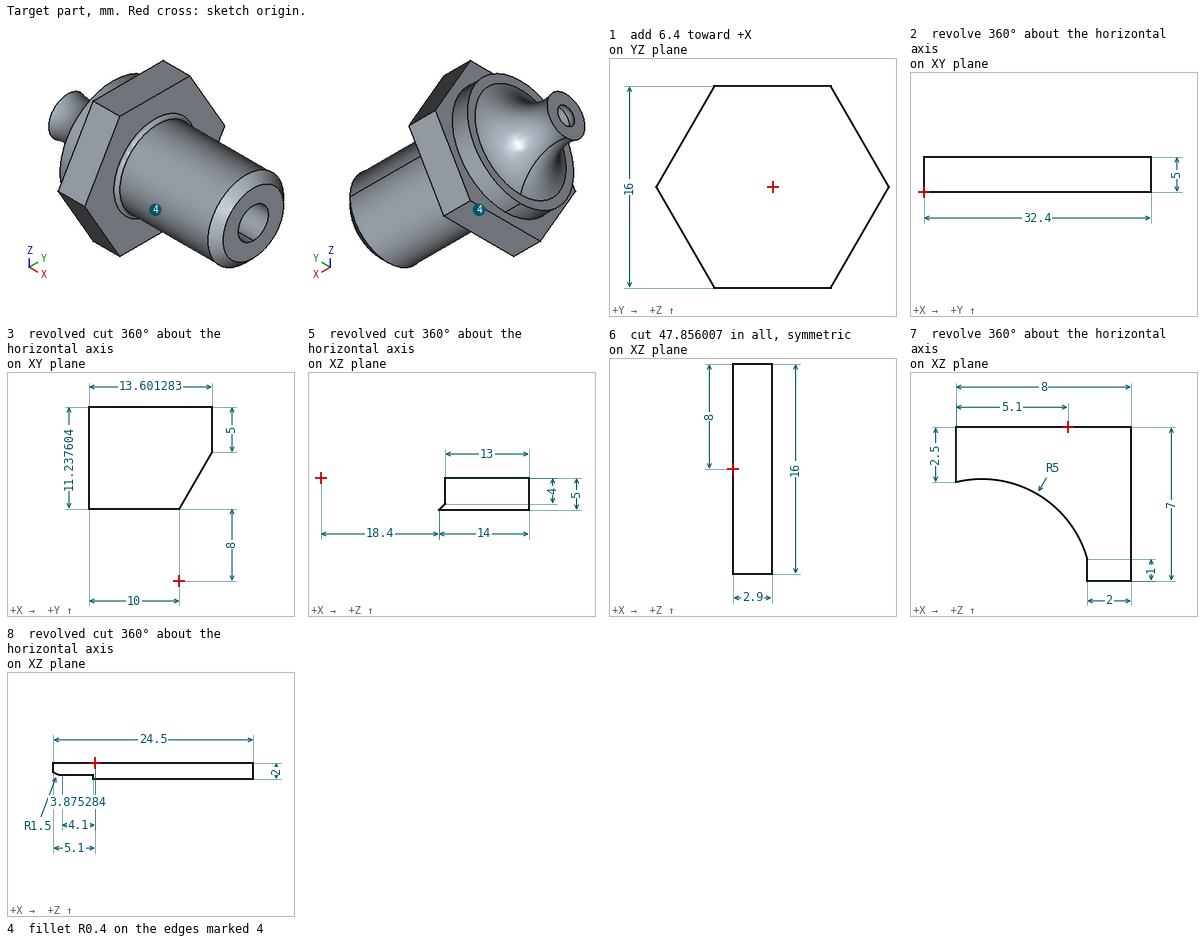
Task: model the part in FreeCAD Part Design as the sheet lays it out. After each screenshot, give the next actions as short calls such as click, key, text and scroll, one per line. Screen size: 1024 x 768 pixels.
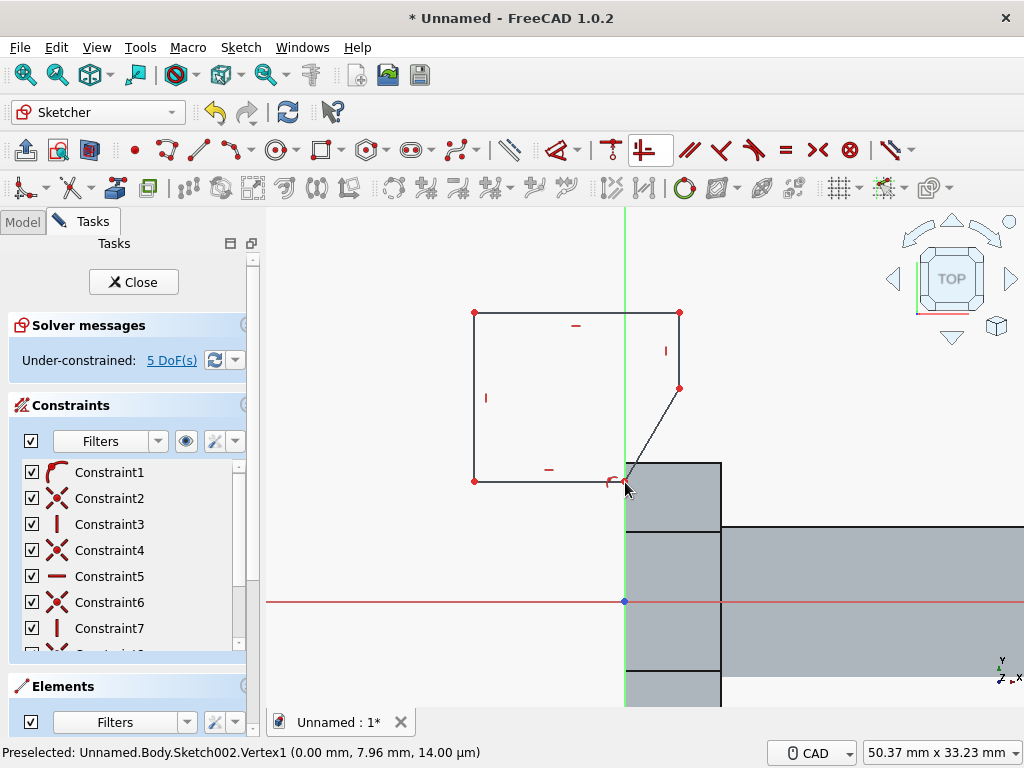
click(556, 150)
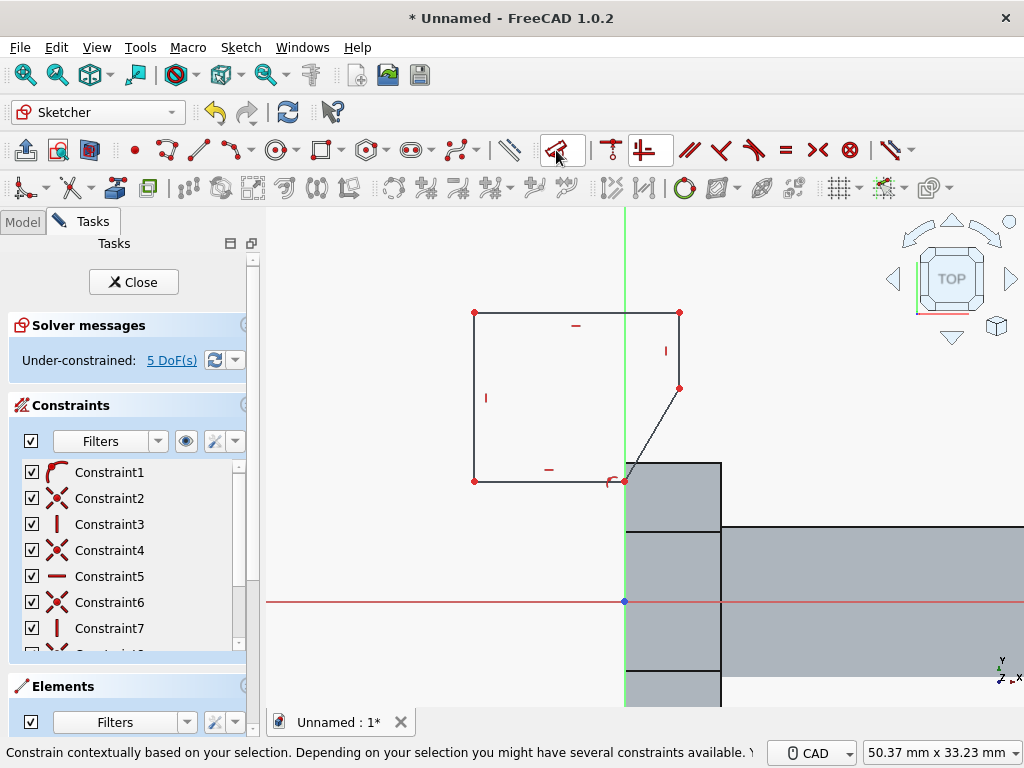
click(679, 366)
click(713, 351)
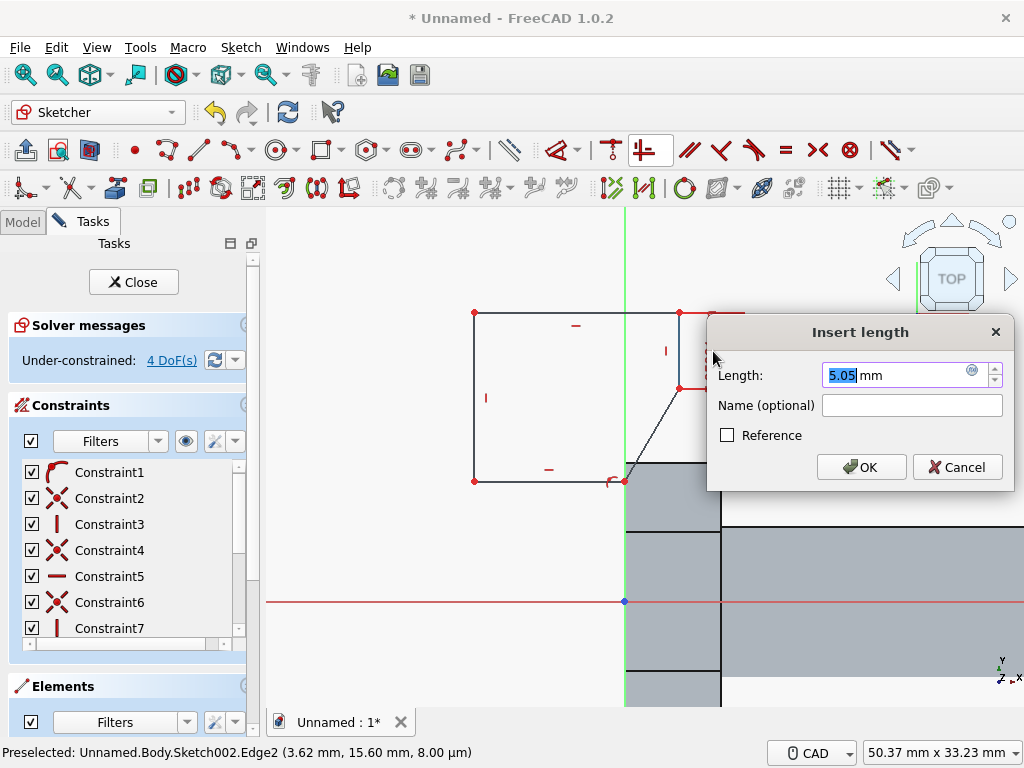
text(5)
key(Return)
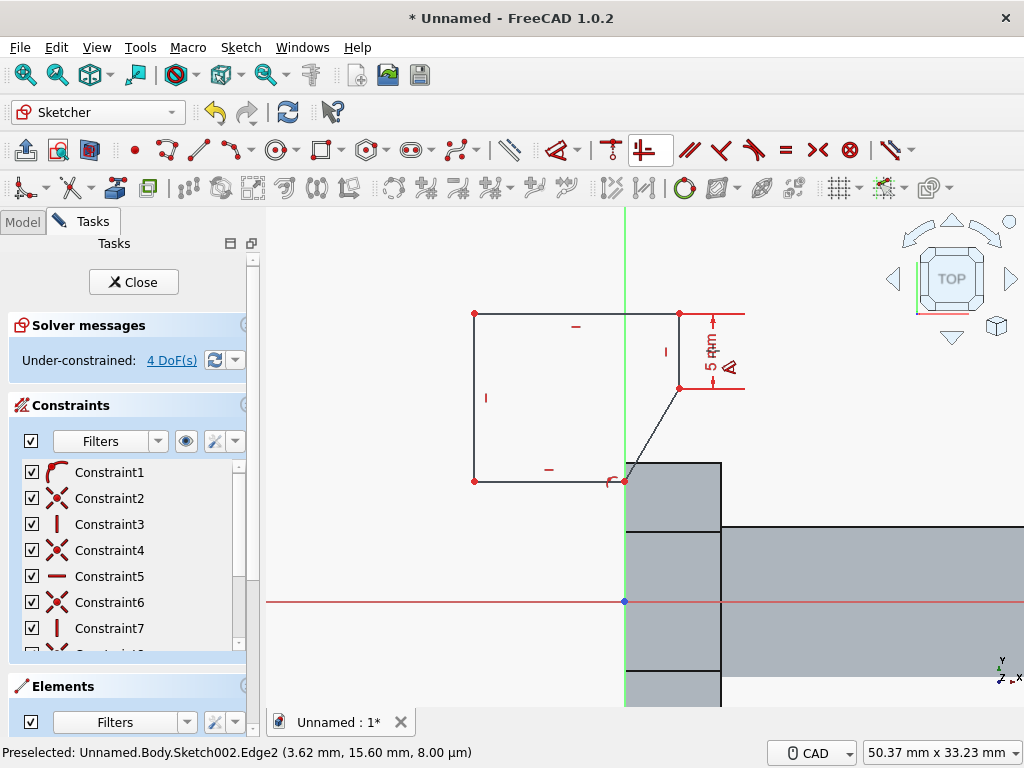
click(519, 482)
click(549, 516)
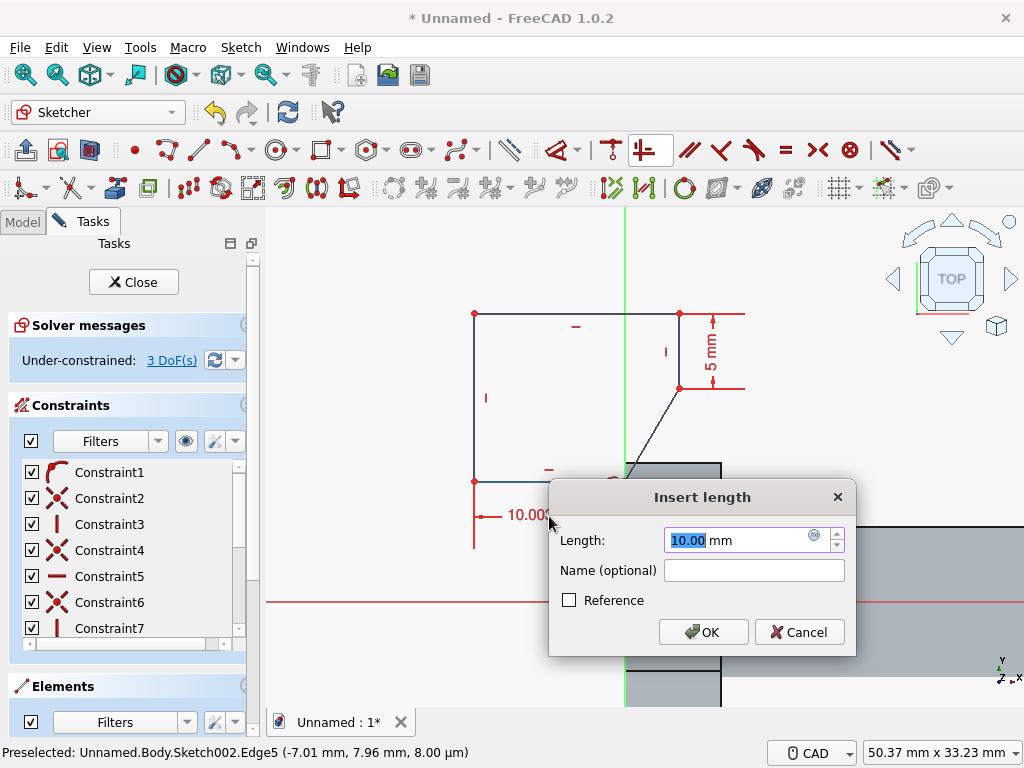
text(10)
key(Return)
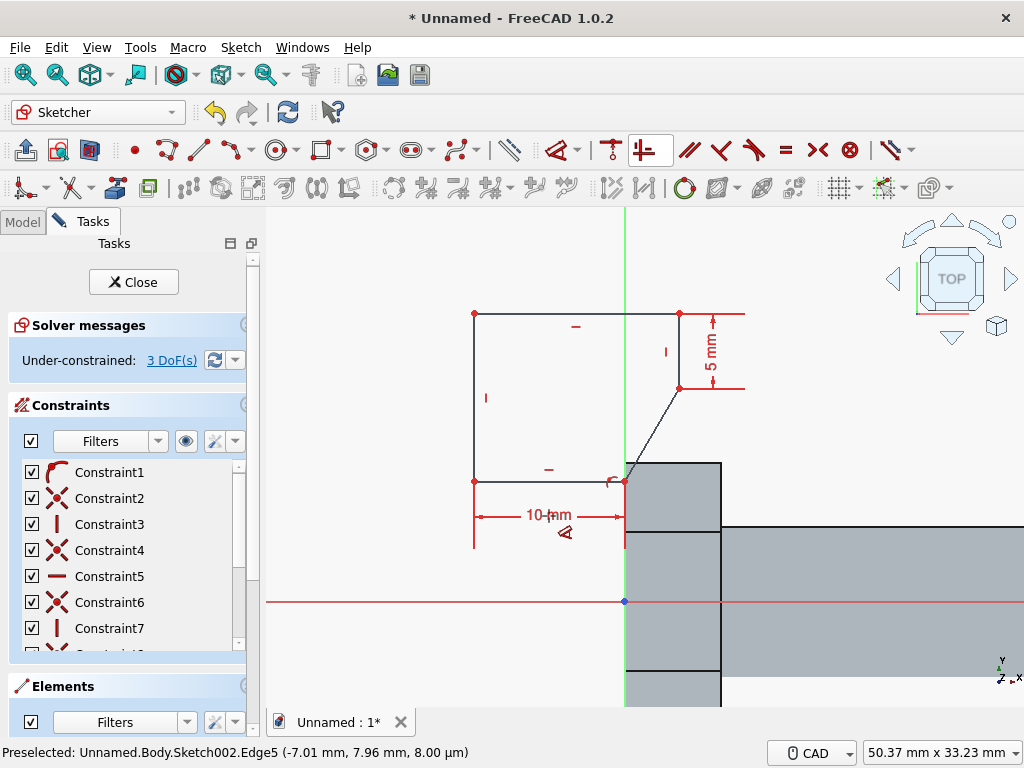
click(625, 482)
click(659, 542)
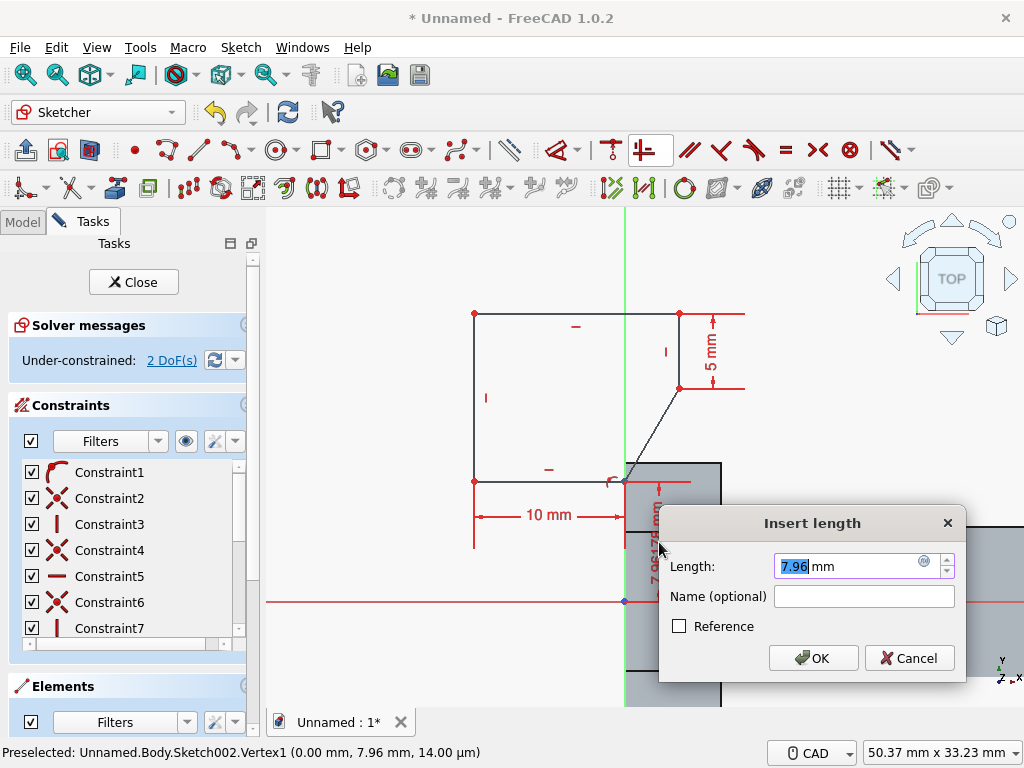
text(8)
key(Return)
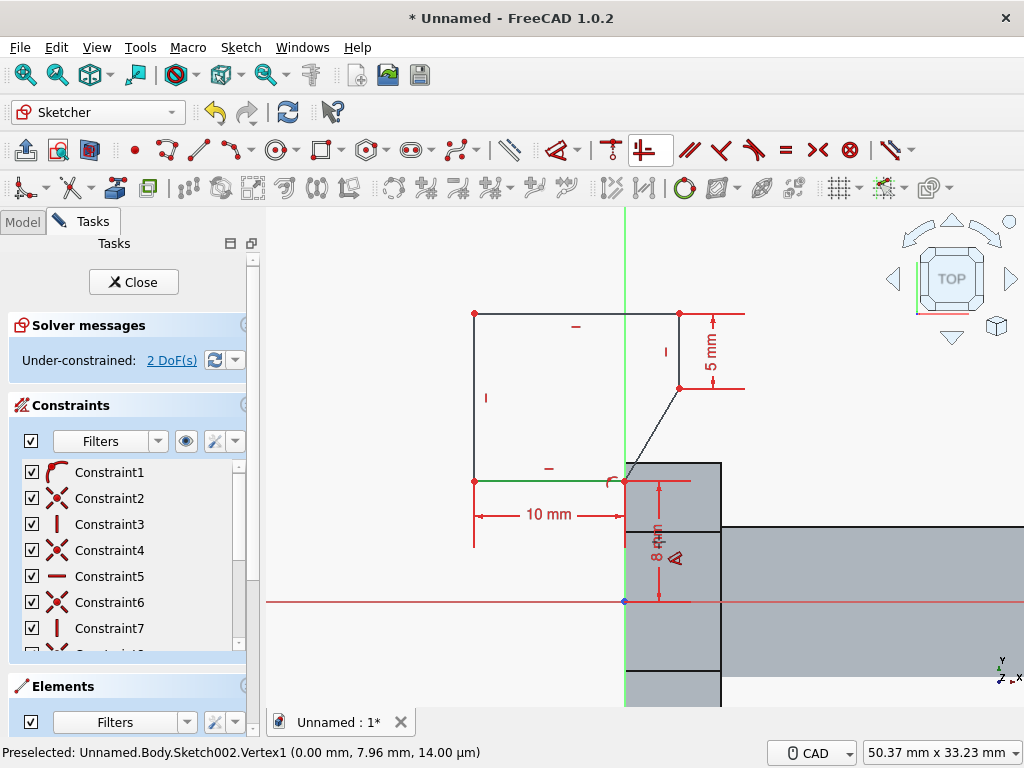
click(536, 314)
click(577, 280)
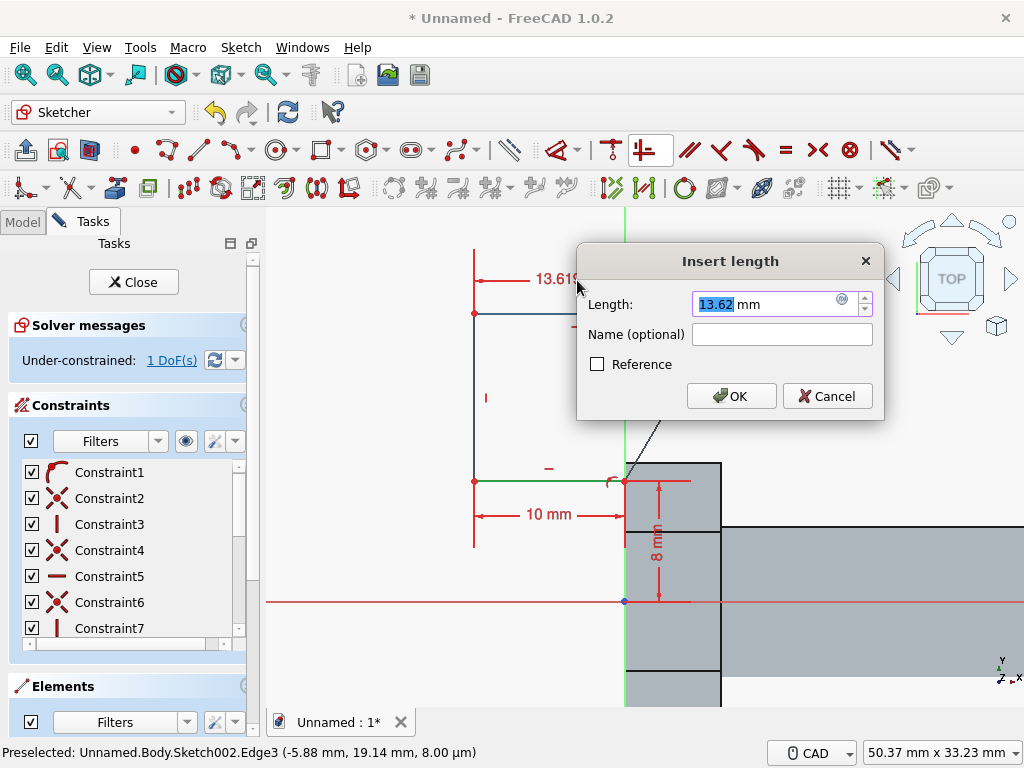
text(13.601283)
key(Return)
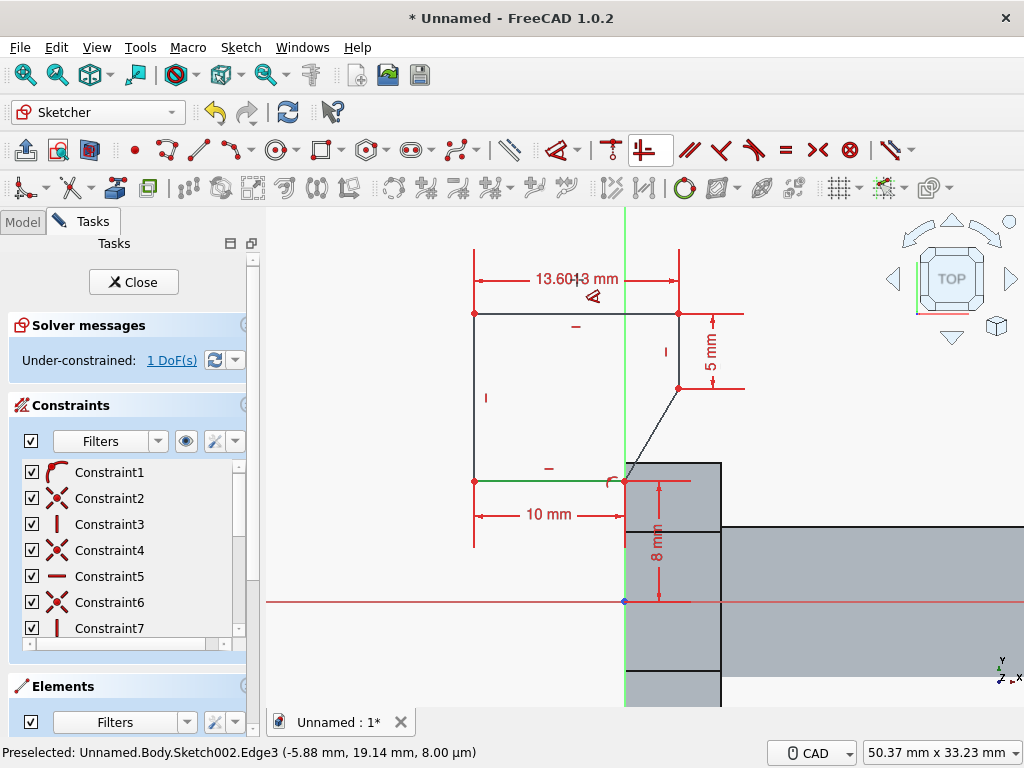
click(474, 364)
click(440, 398)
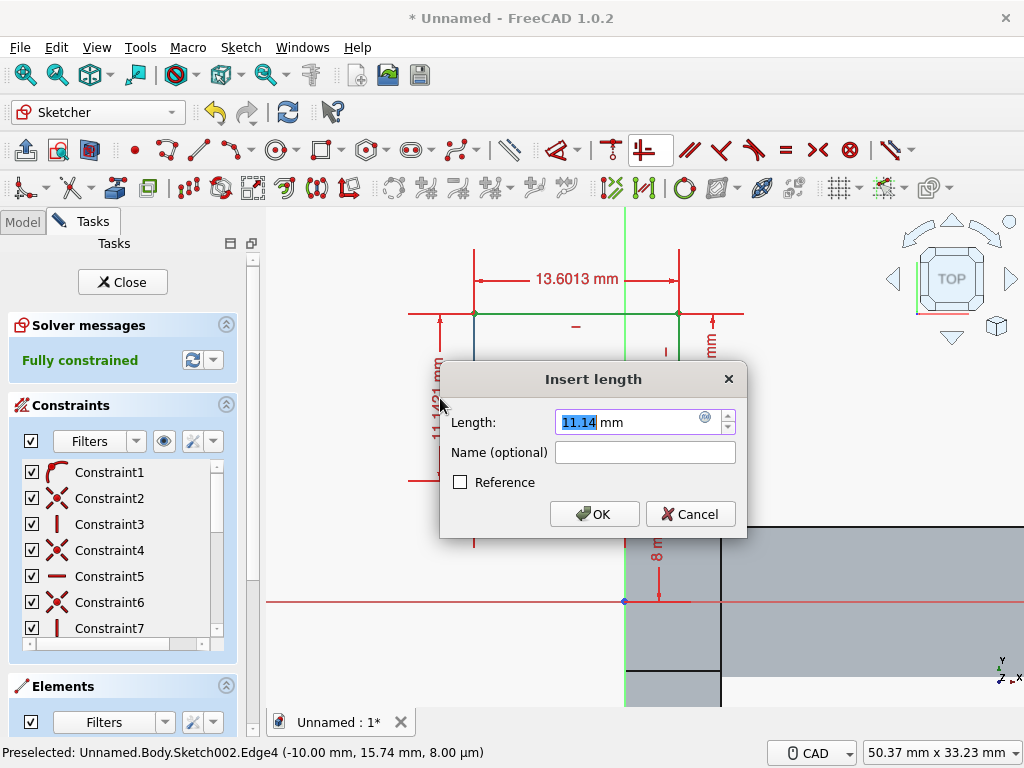
text(11.237604)
key(Return)
key(Escape)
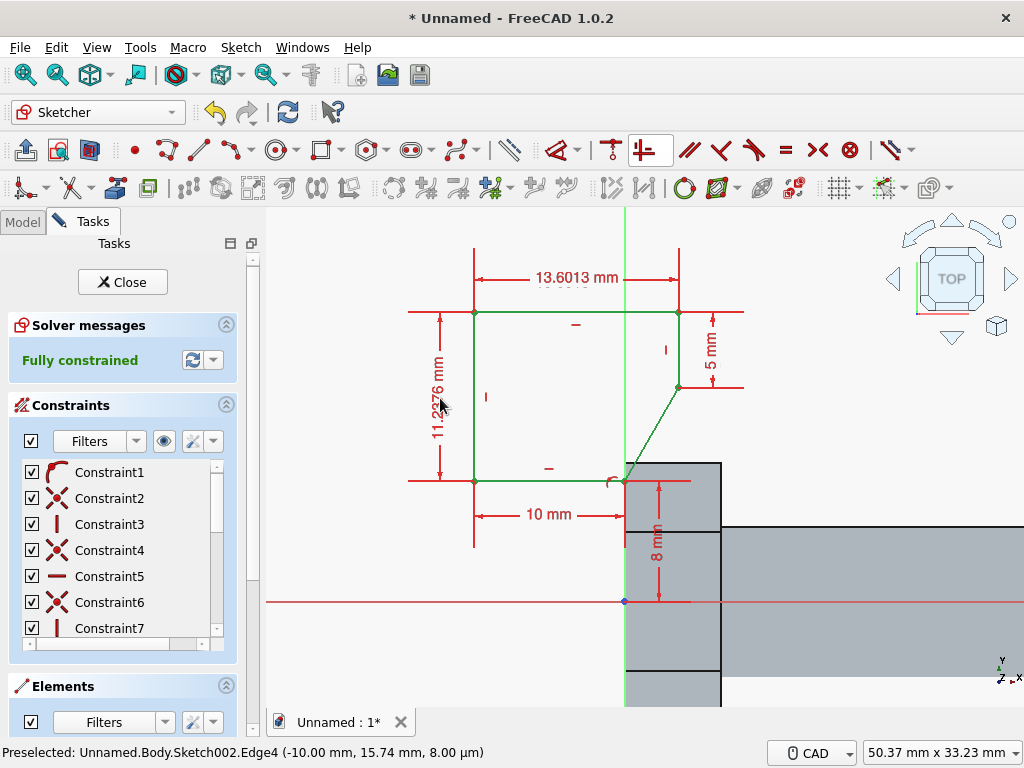
click(123, 282)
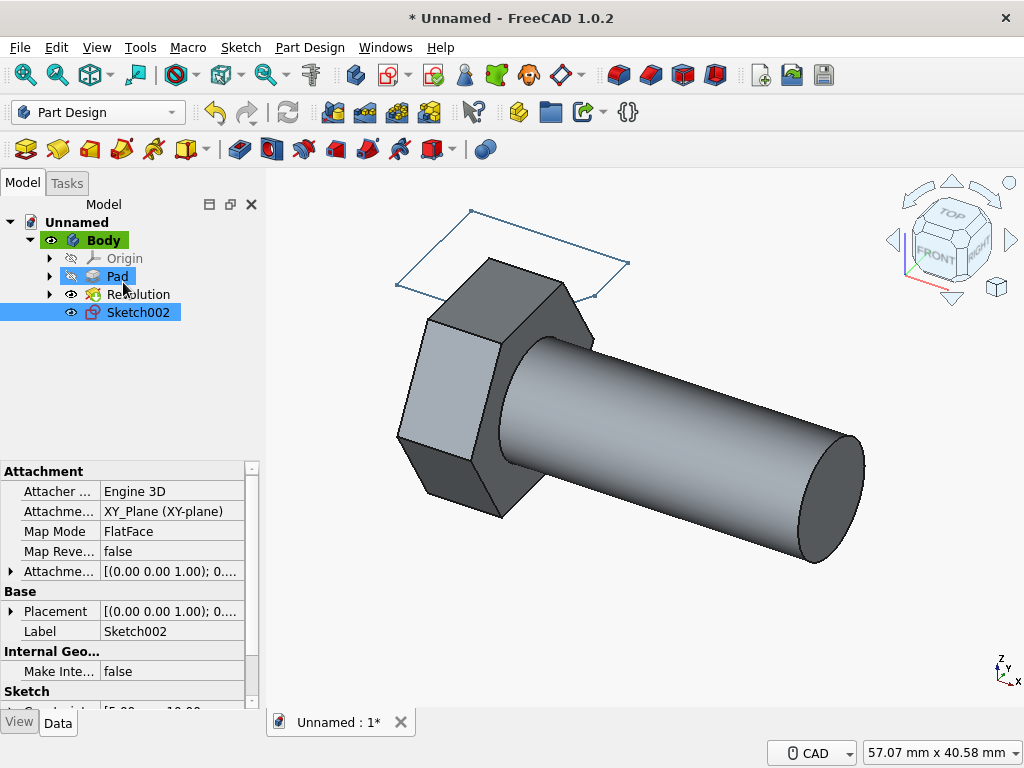
click(304, 150)